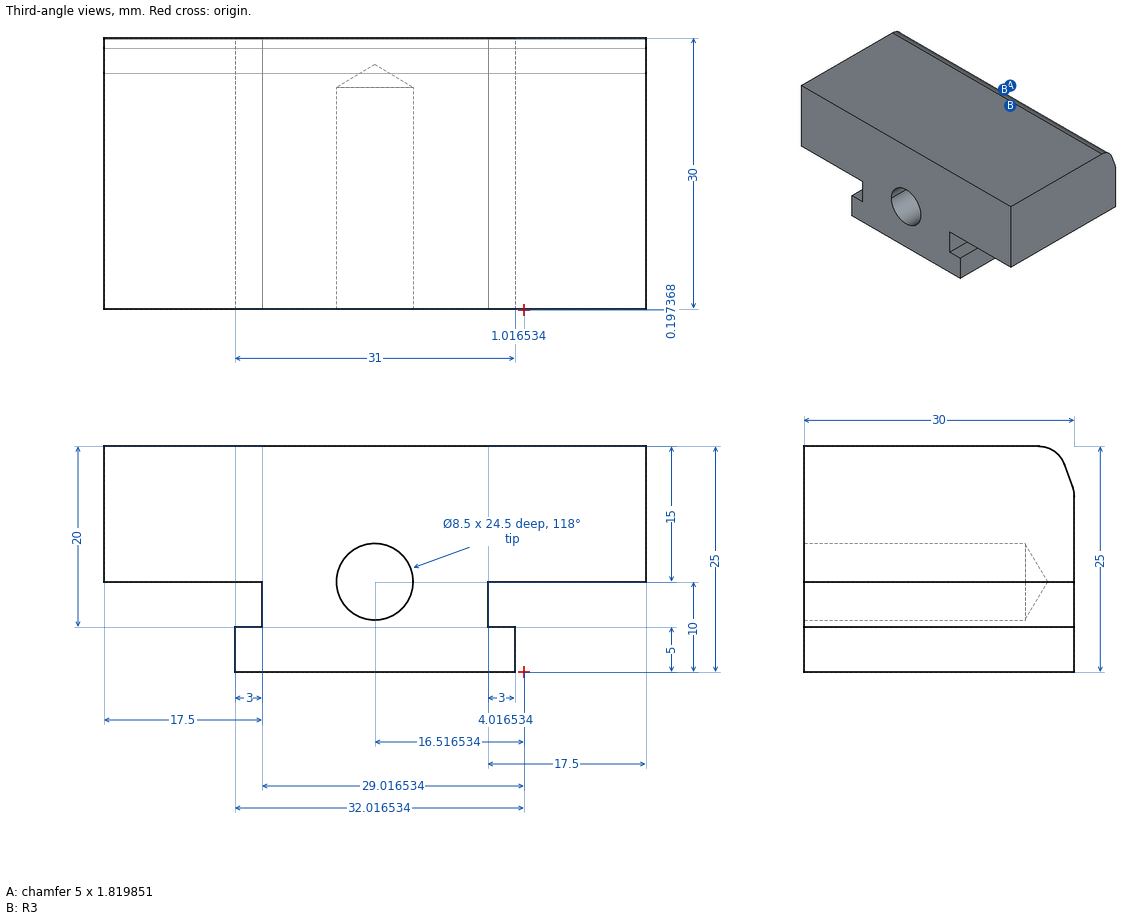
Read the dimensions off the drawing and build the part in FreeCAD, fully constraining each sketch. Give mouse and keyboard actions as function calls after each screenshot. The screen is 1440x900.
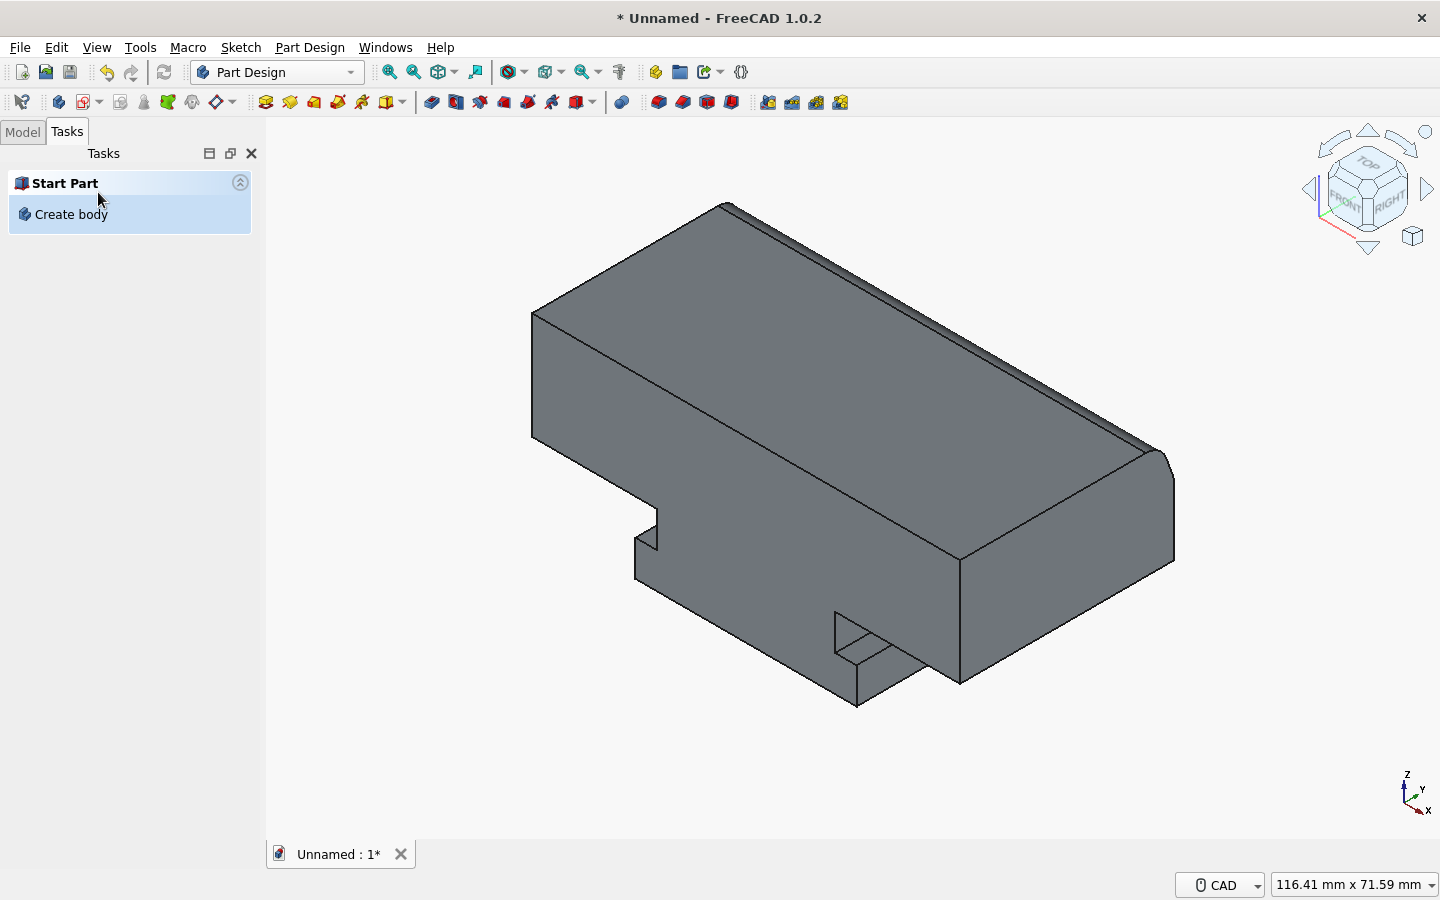
click(746, 539)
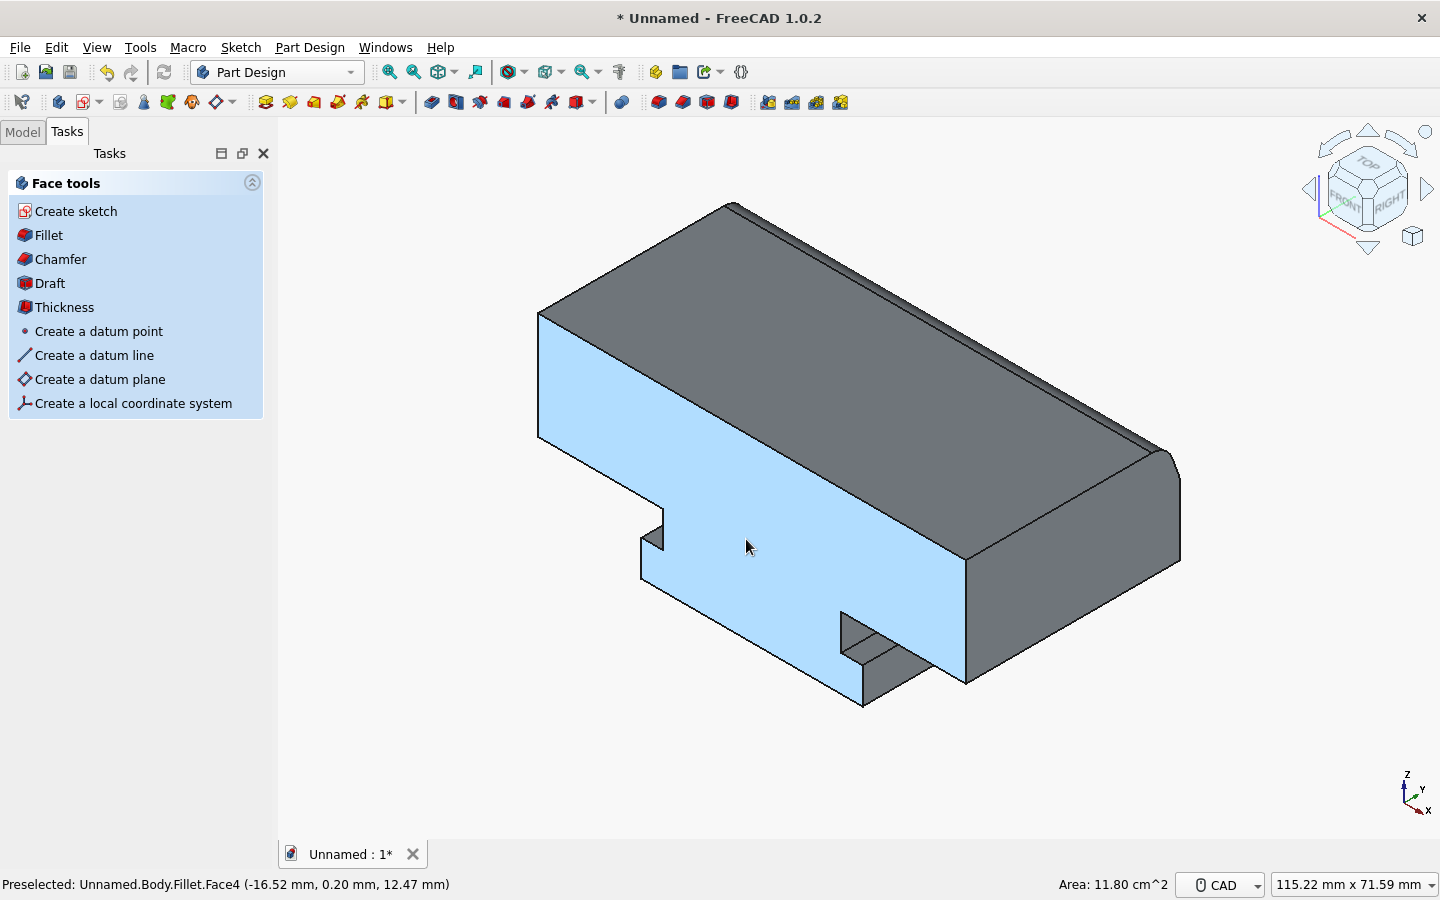
click(84, 102)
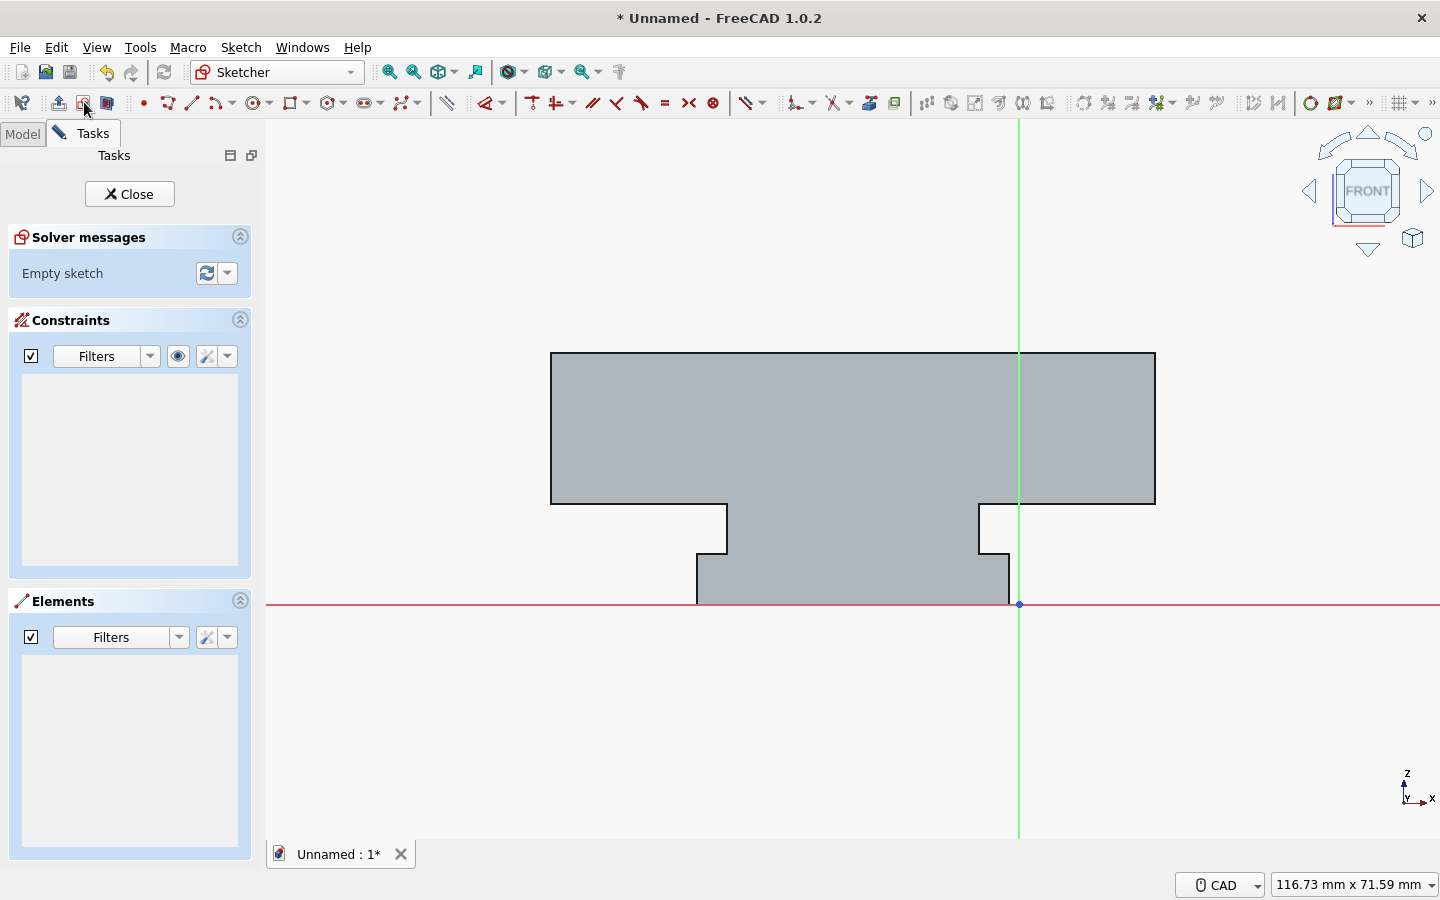
scroll(971, 556, up, 6)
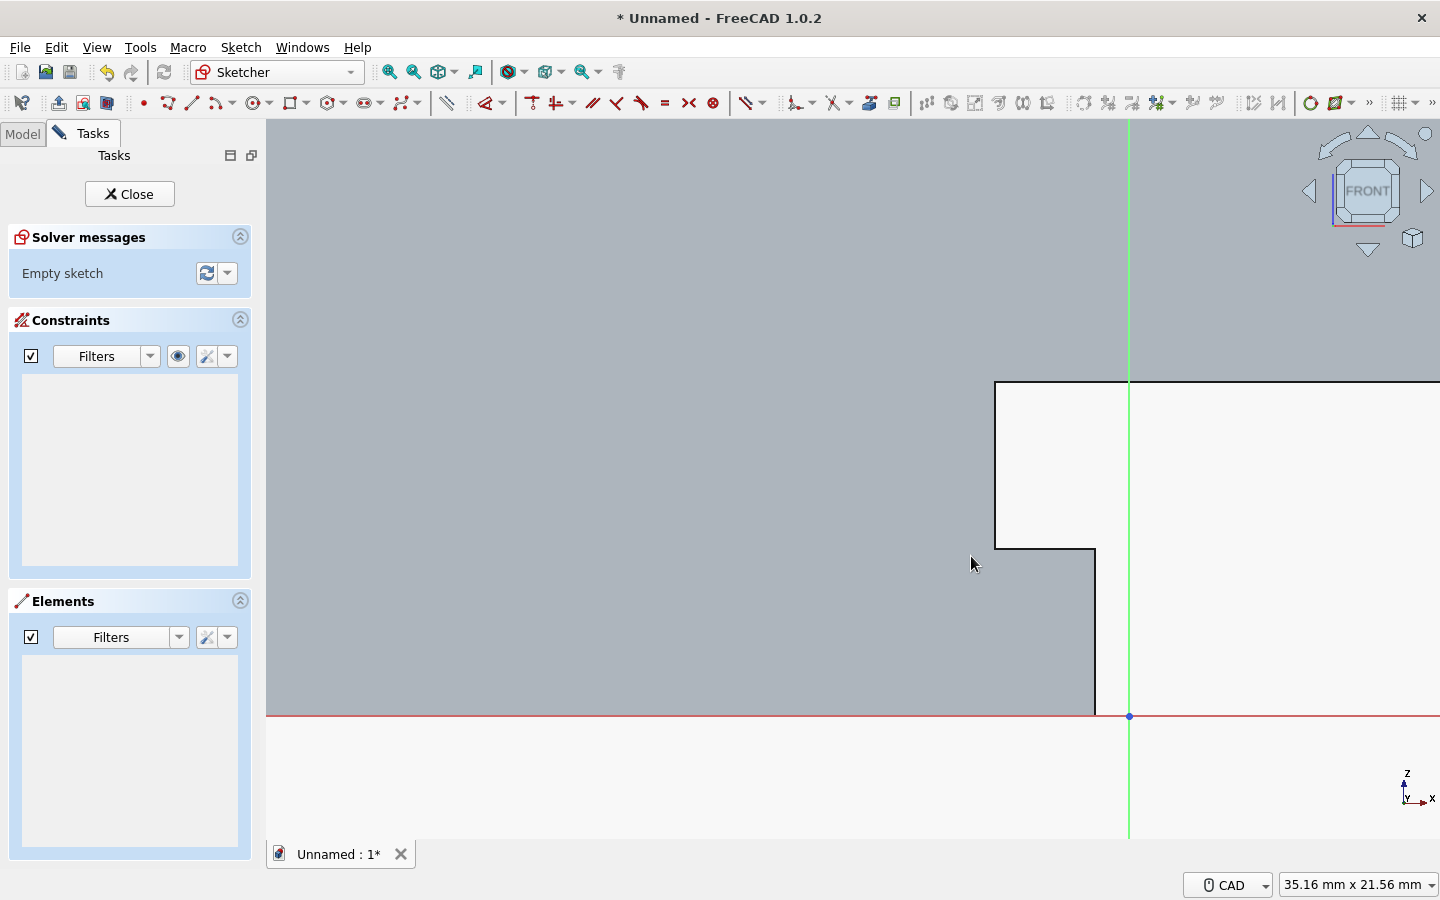
click(254, 104)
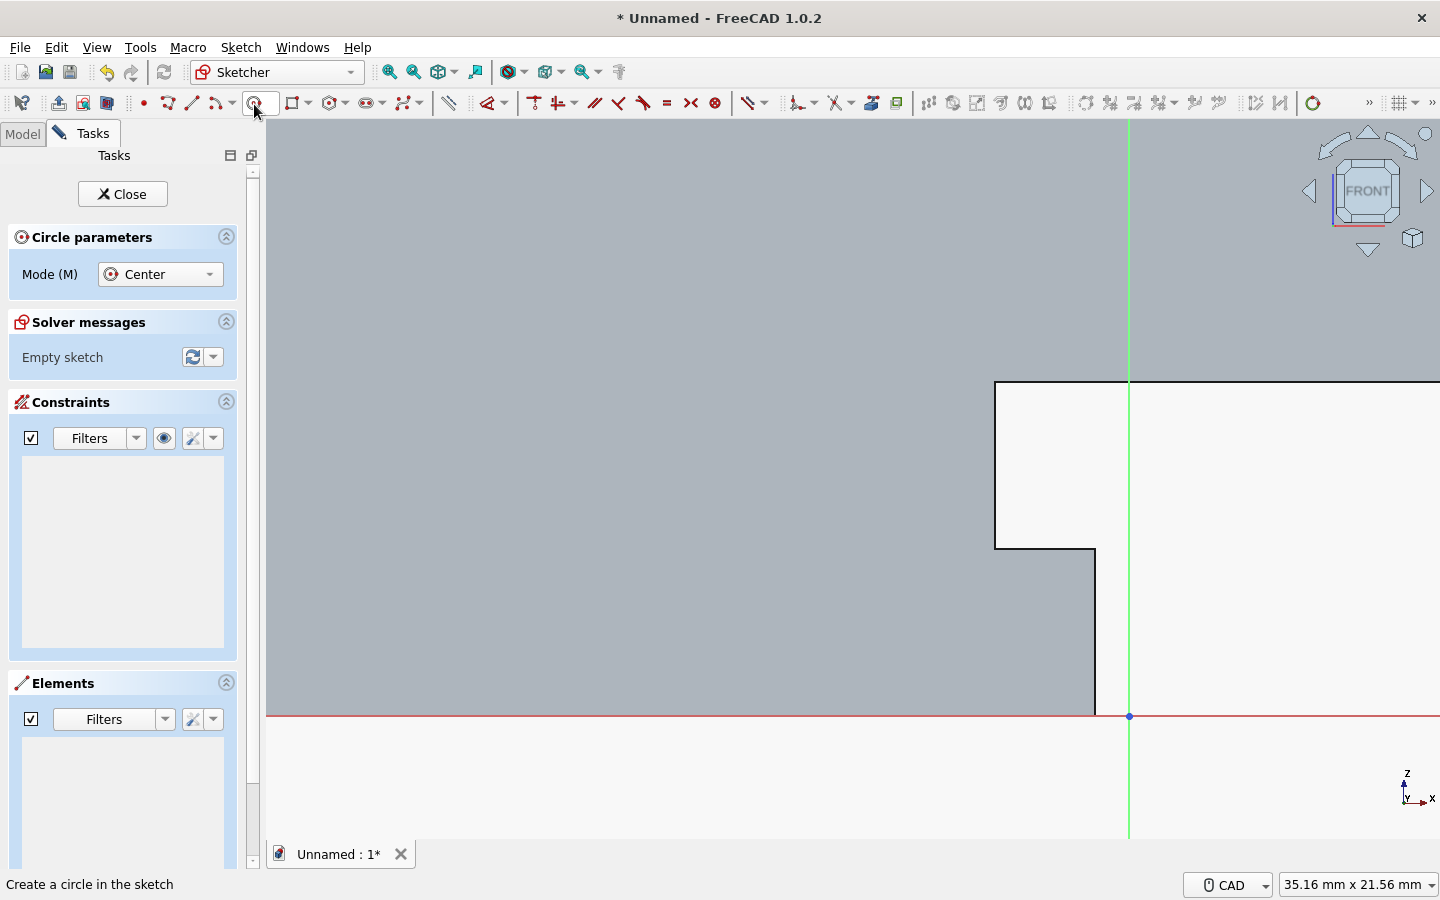
click(578, 382)
move(678, 282)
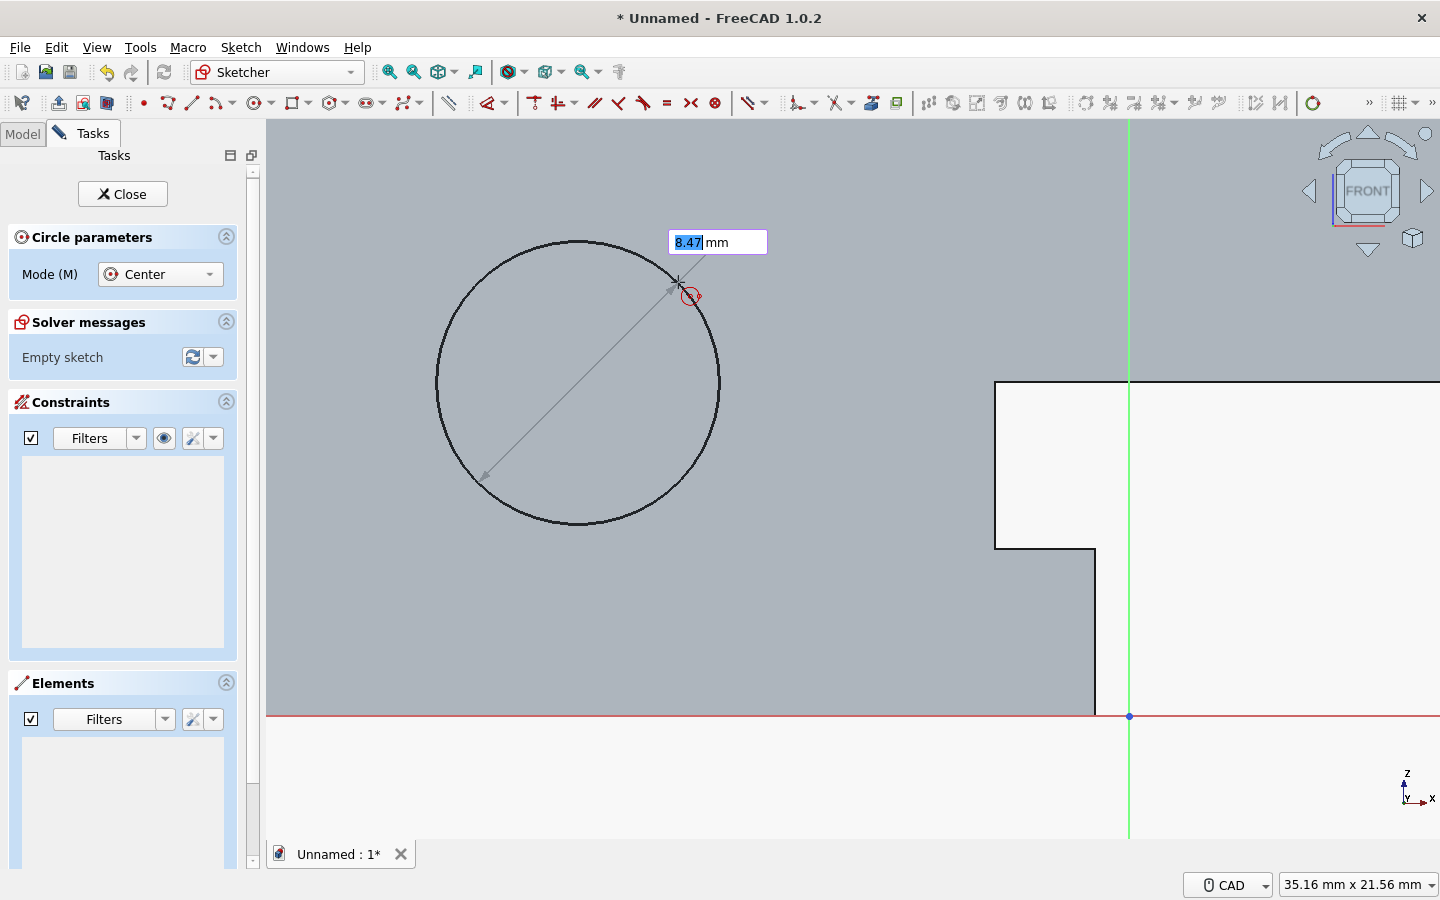
text(8.5)
key(Return)
key(Escape)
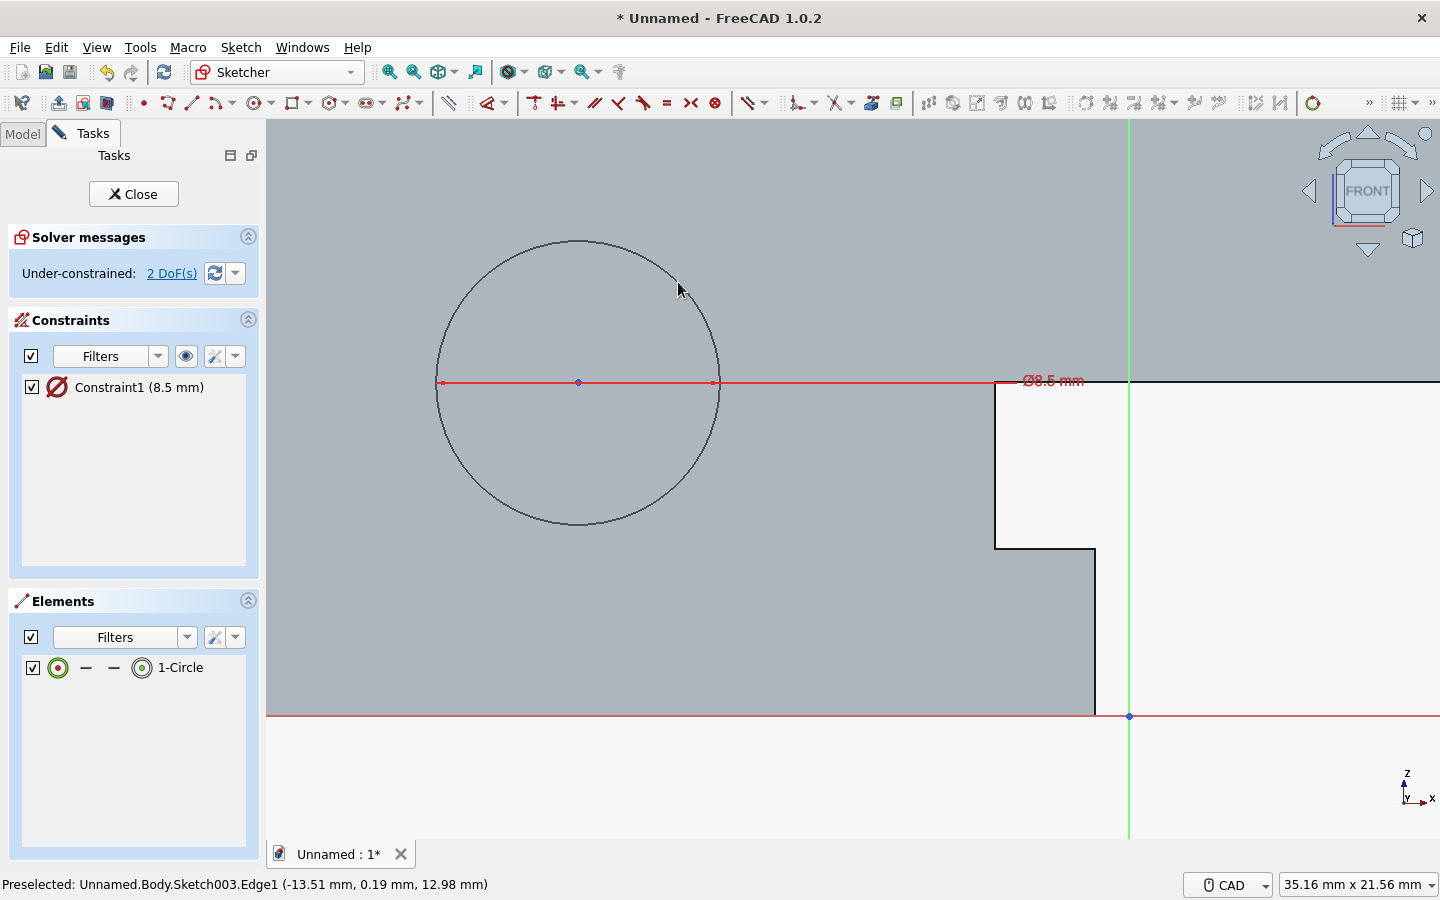
click(488, 104)